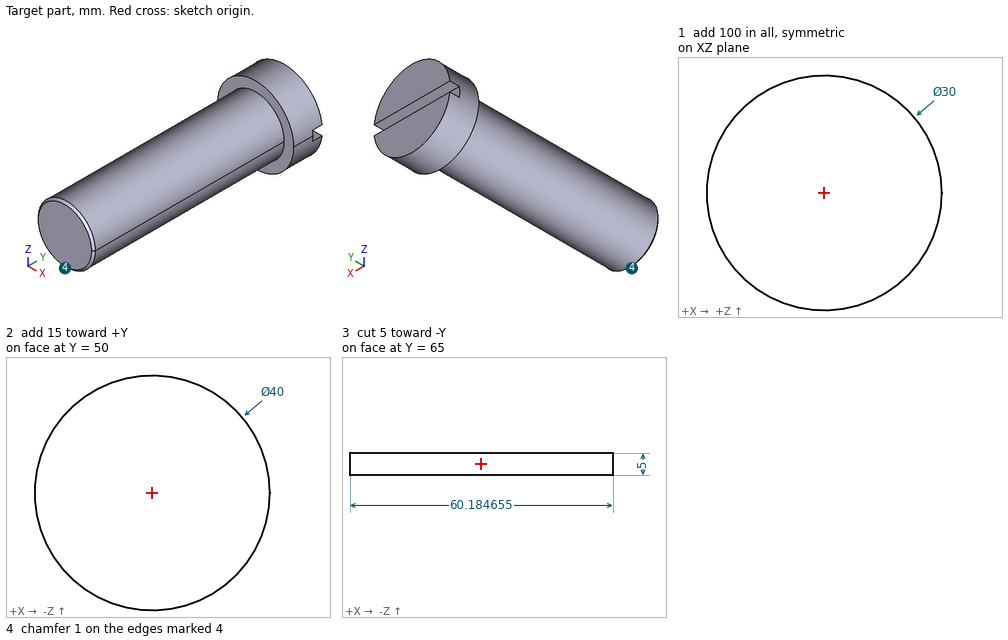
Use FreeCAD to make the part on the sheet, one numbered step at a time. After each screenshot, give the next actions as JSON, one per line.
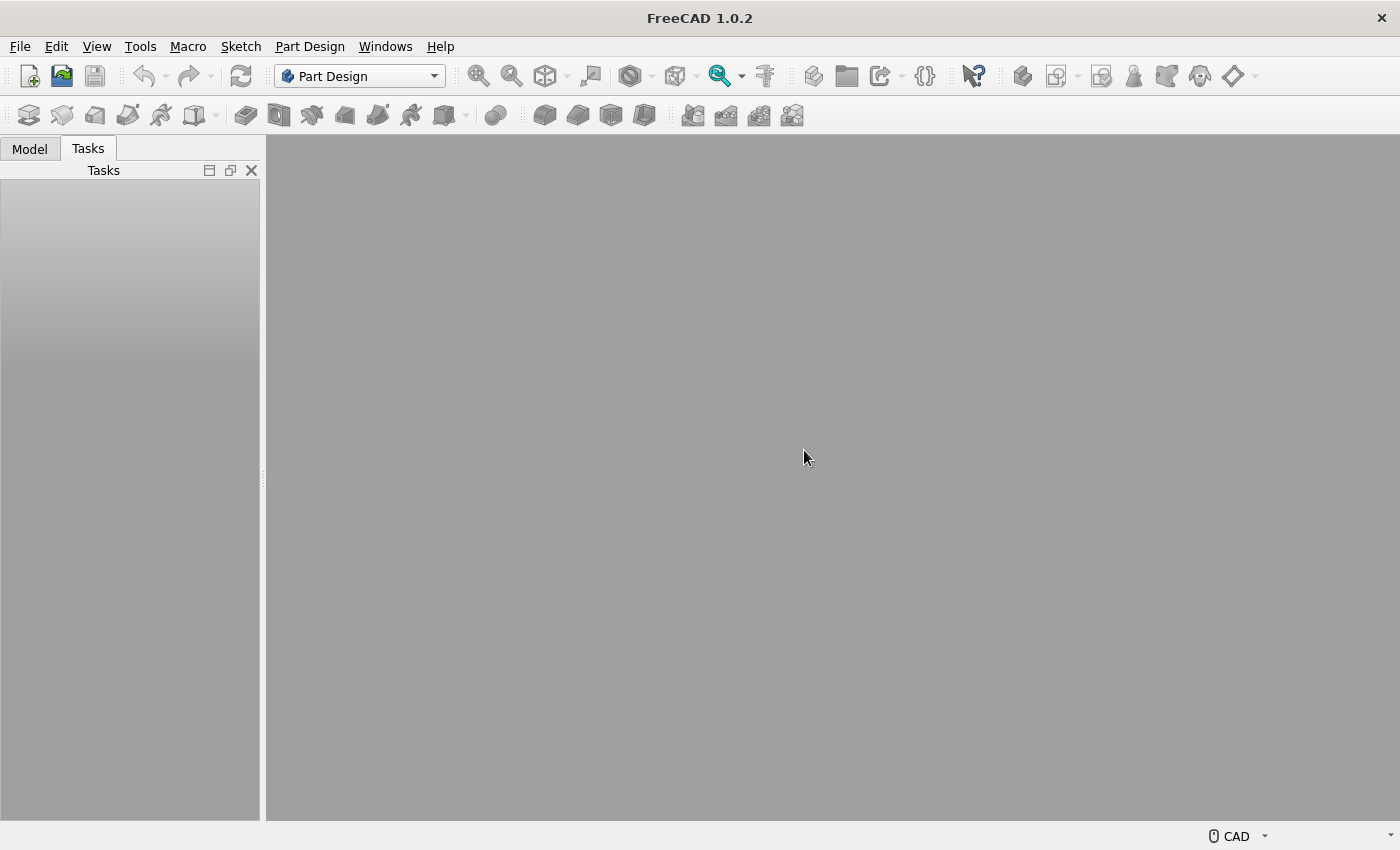
{"action": "left_click", "coordinate": [29, 76]}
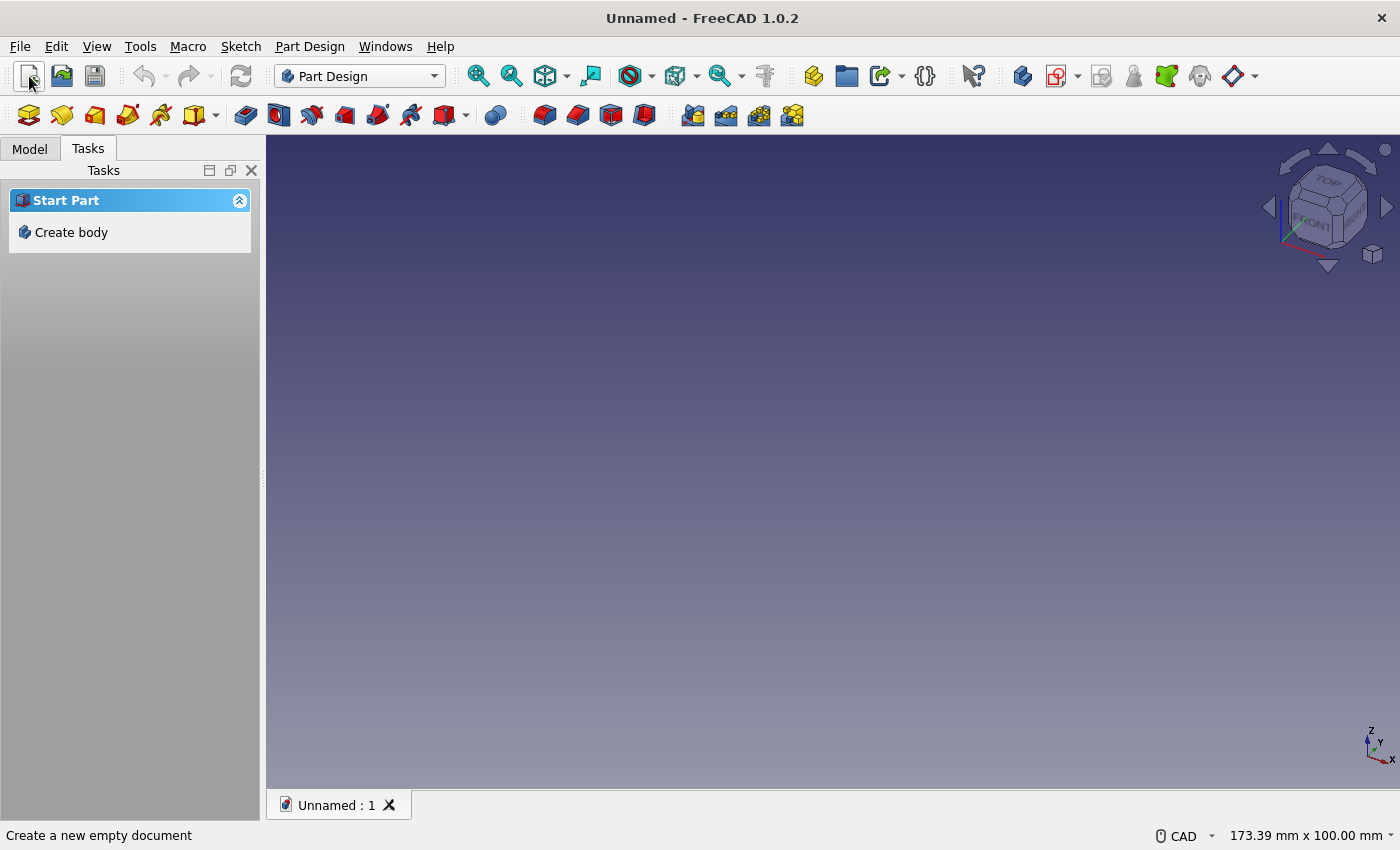
{"action": "left_click", "coordinate": [1056, 76]}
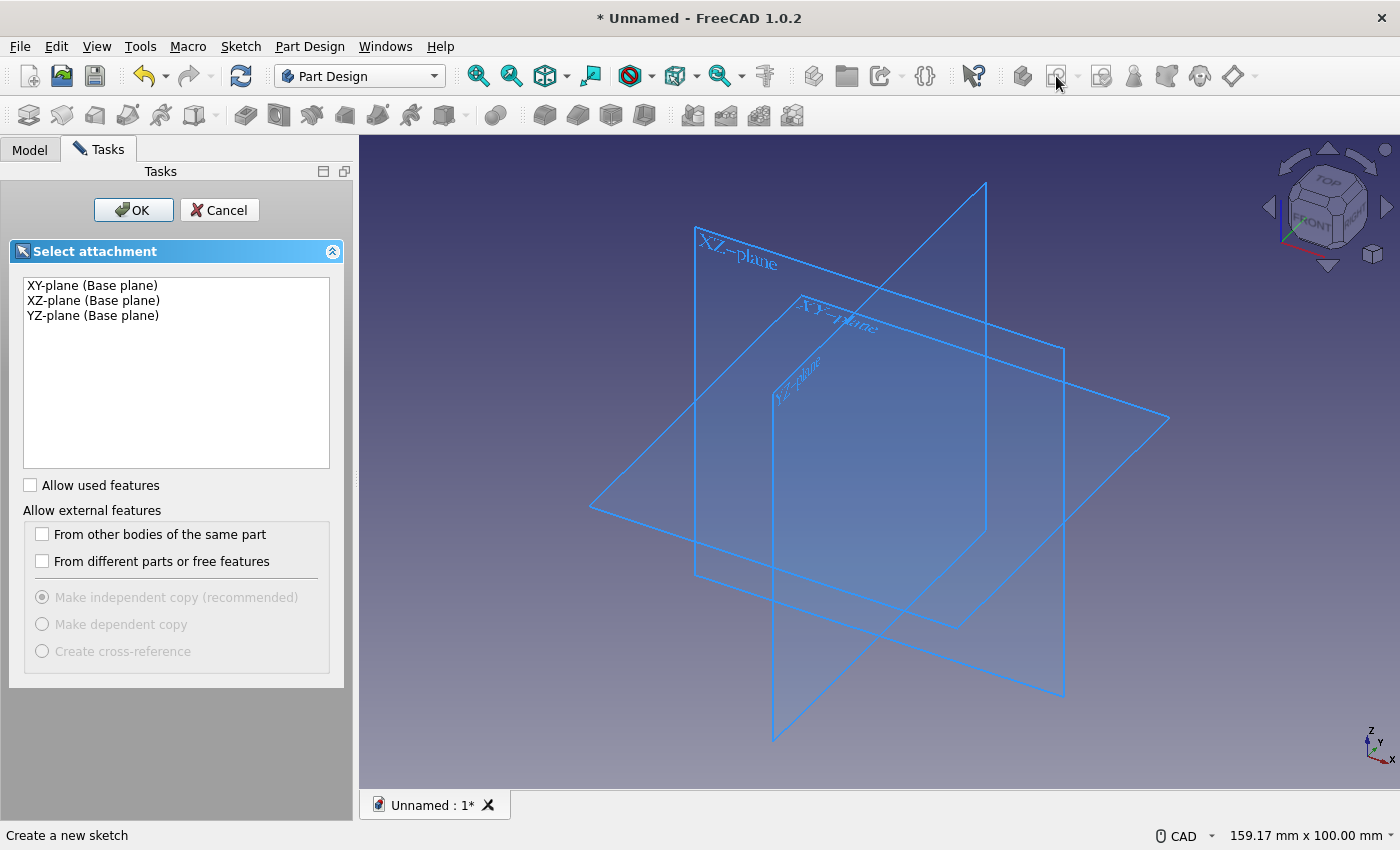
{"action": "left_click", "coordinate": [84, 300]}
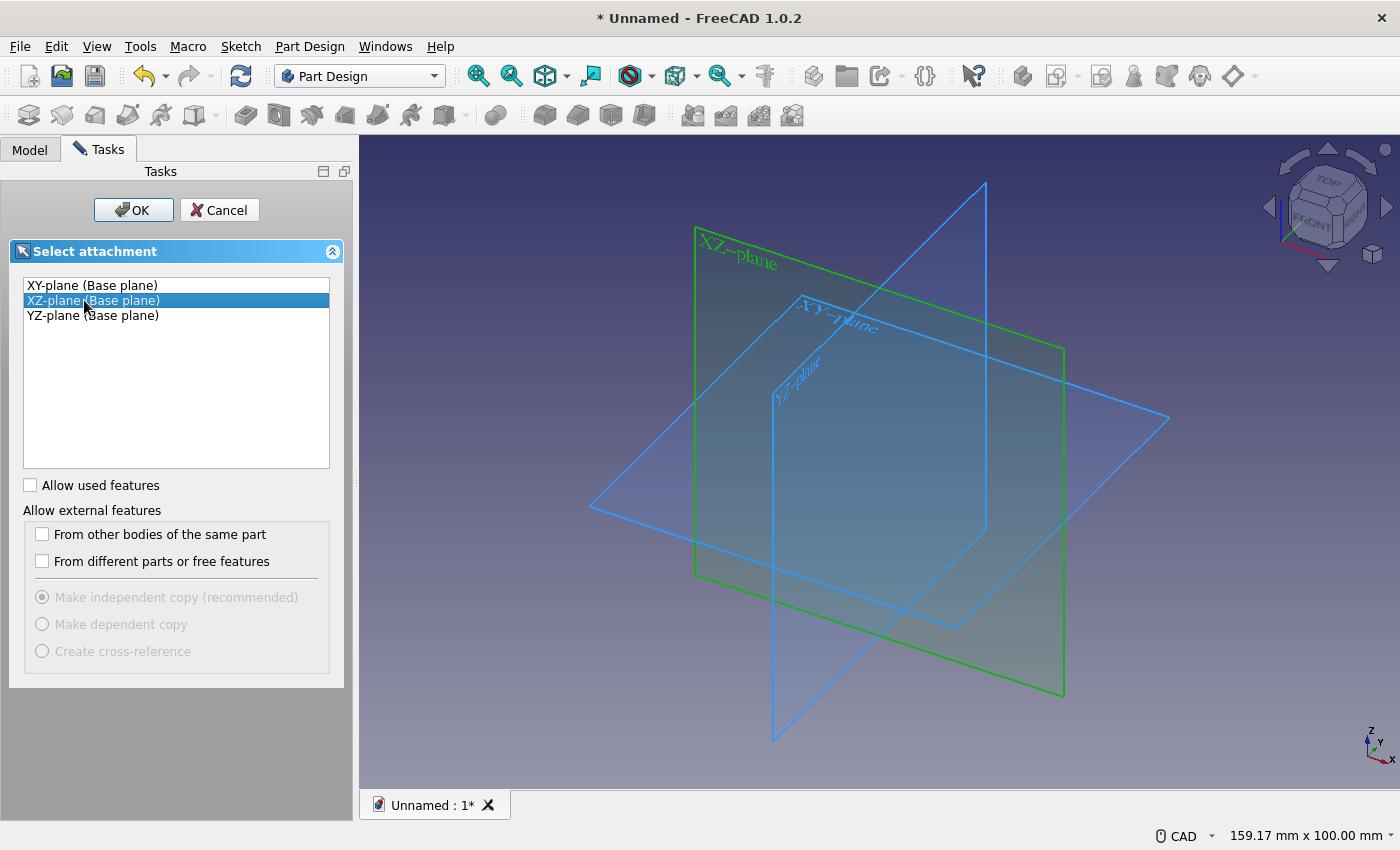
{"action": "left_click", "coordinate": [134, 210]}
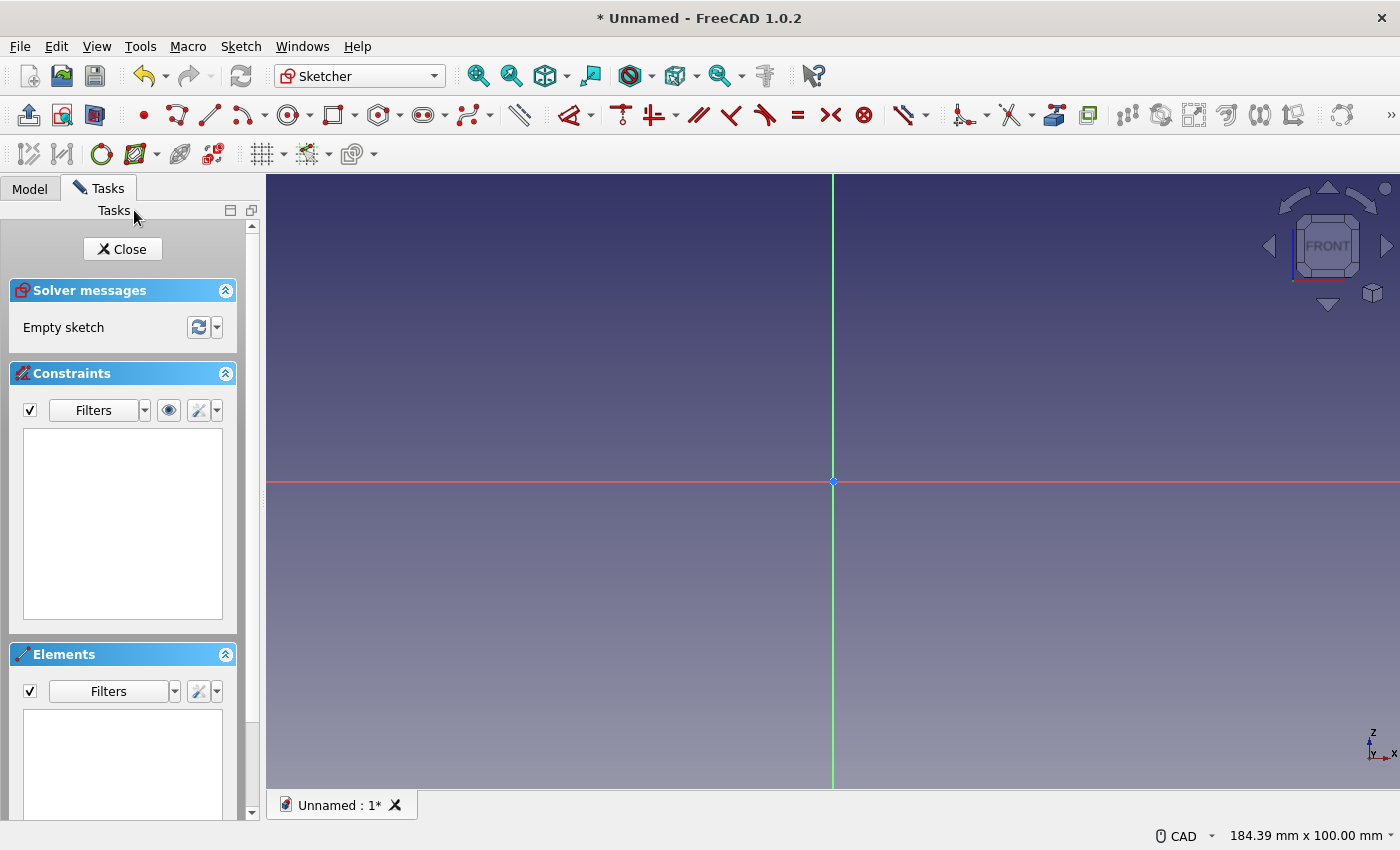
{"action": "scroll", "coordinate": [889, 482], "scroll_direction": "up", "scroll_amount": 4}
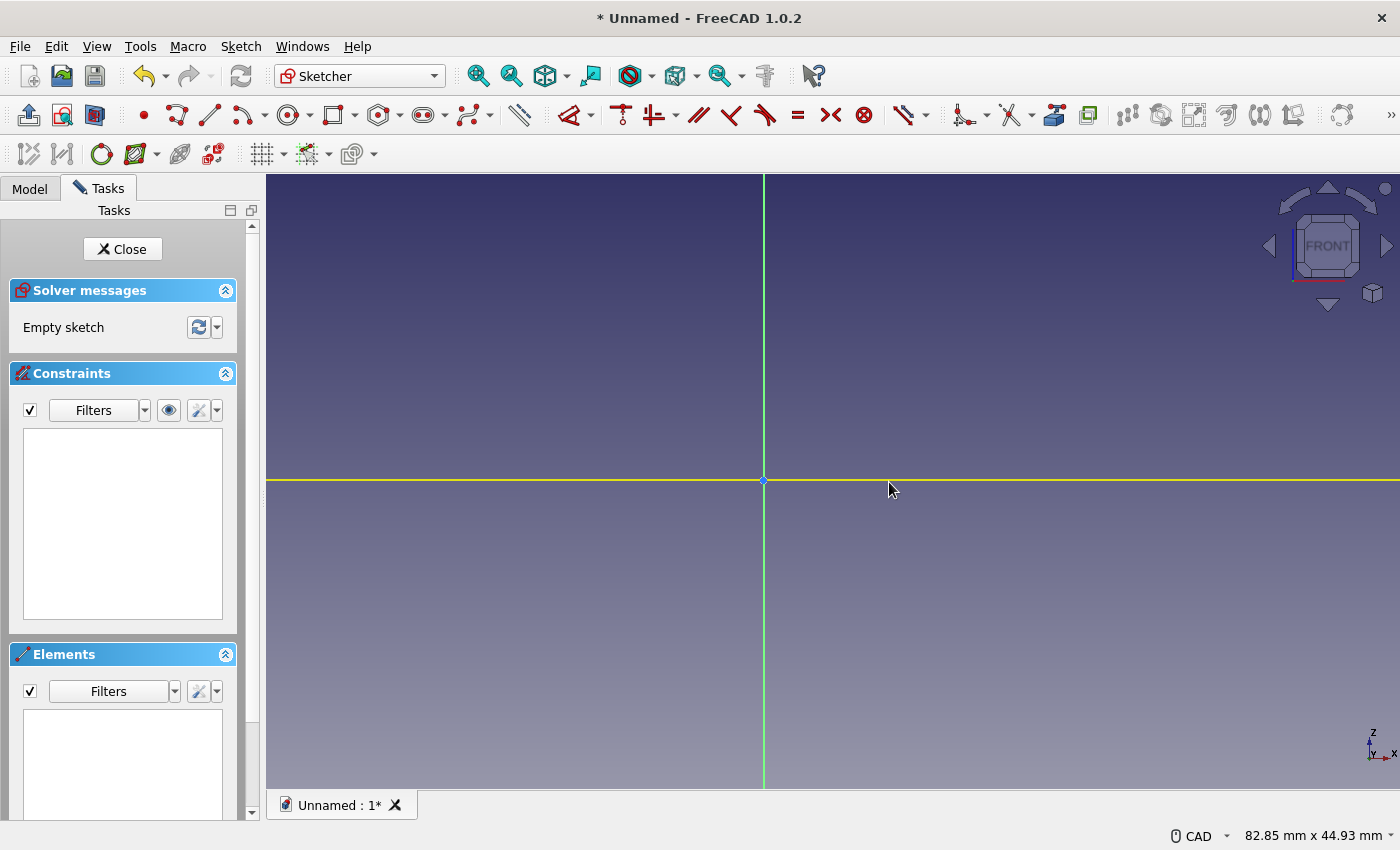
{"action": "left_click", "coordinate": [288, 116]}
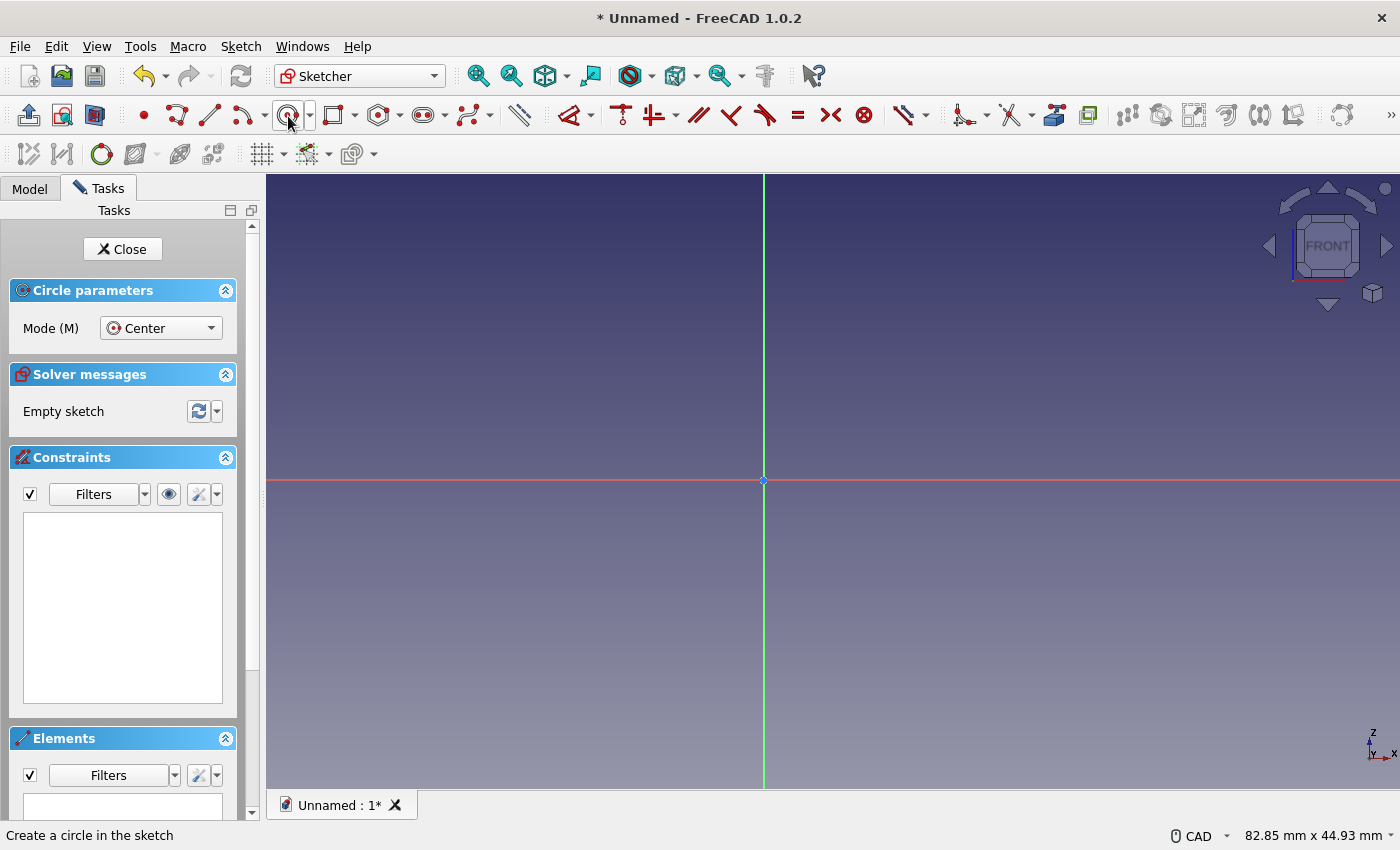
{"action": "left_click", "coordinate": [764, 480]}
{"action": "left_click", "coordinate": [909, 335]}
{"action": "key", "text": "Escape"}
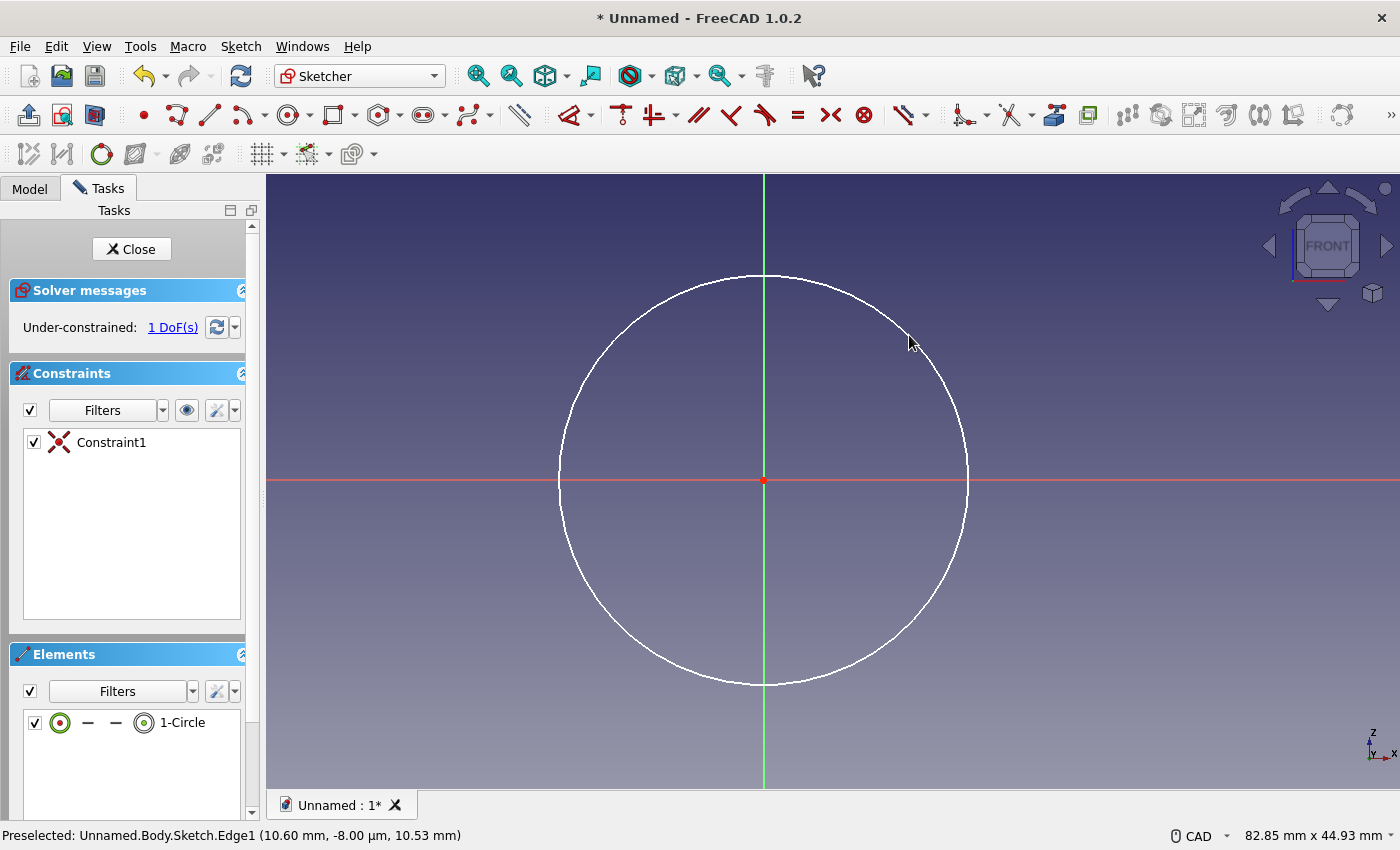
{"action": "left_click", "coordinate": [568, 116]}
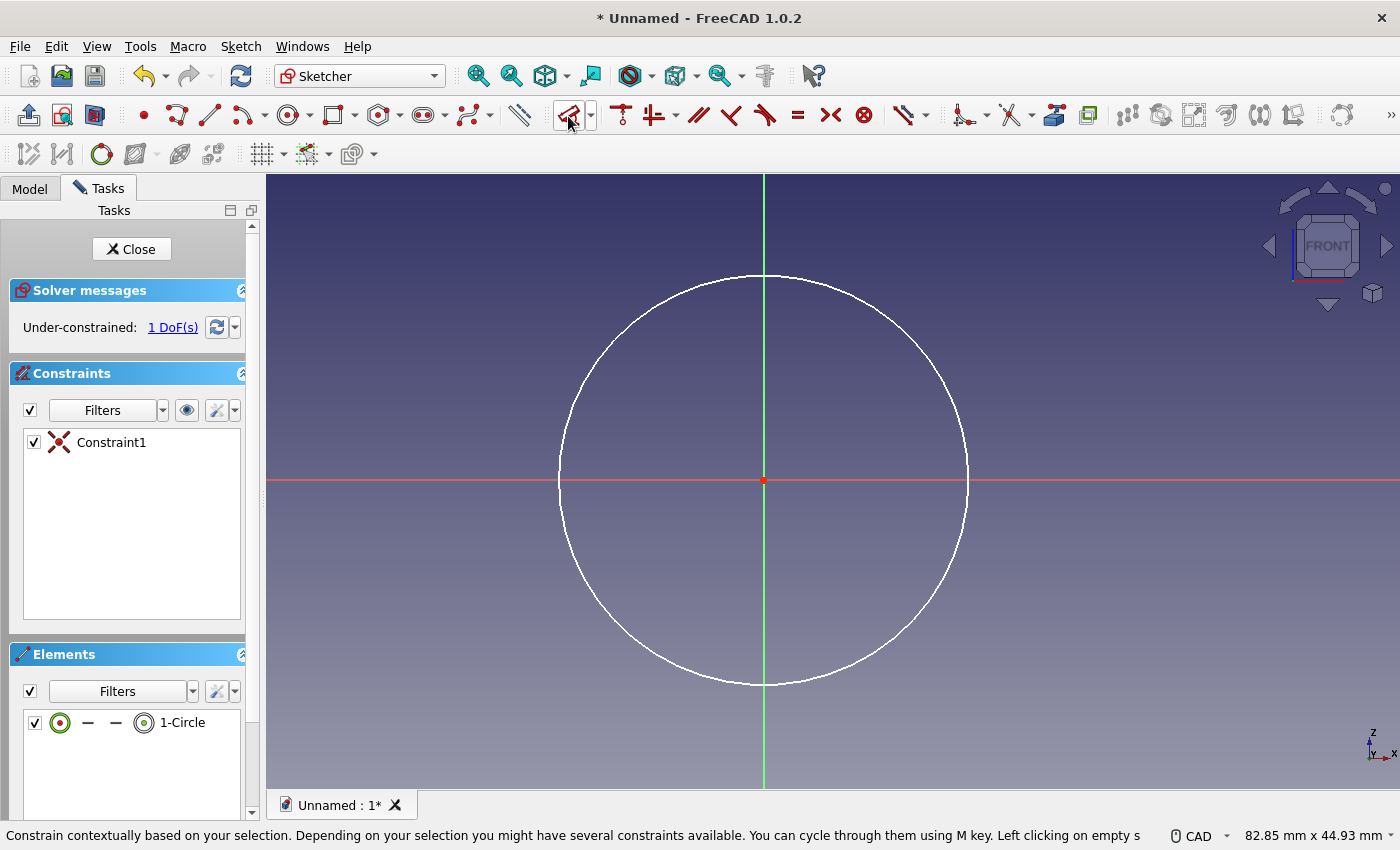
{"action": "left_click", "coordinate": [908, 335]}
{"action": "left_click", "coordinate": [931, 312]}